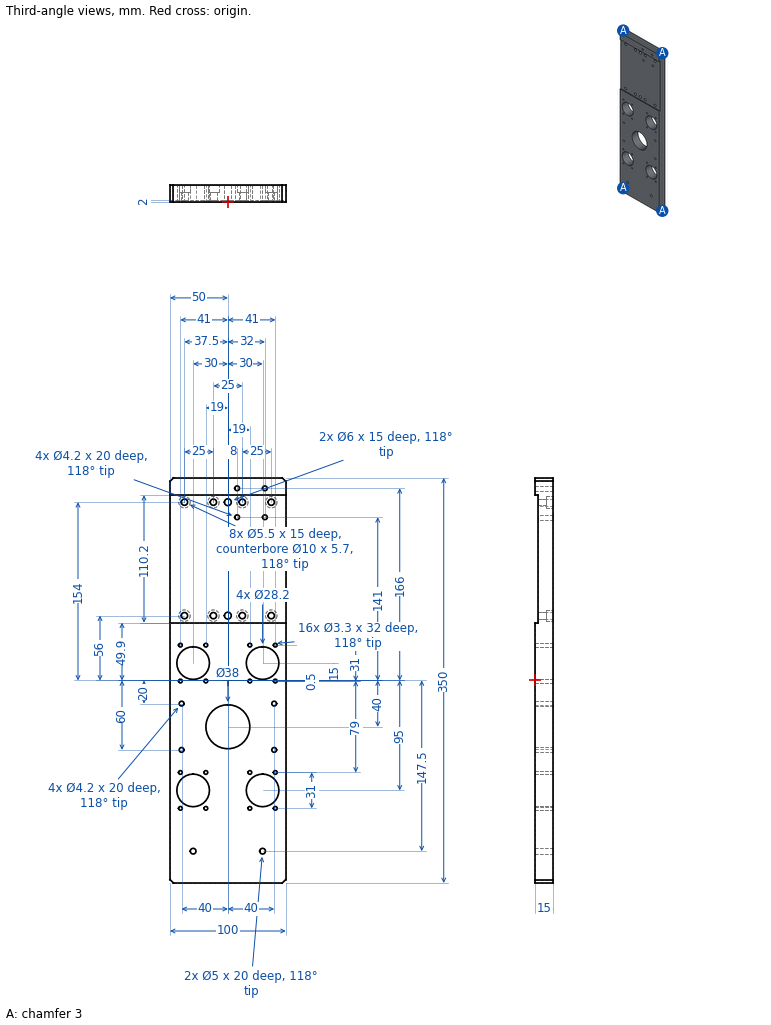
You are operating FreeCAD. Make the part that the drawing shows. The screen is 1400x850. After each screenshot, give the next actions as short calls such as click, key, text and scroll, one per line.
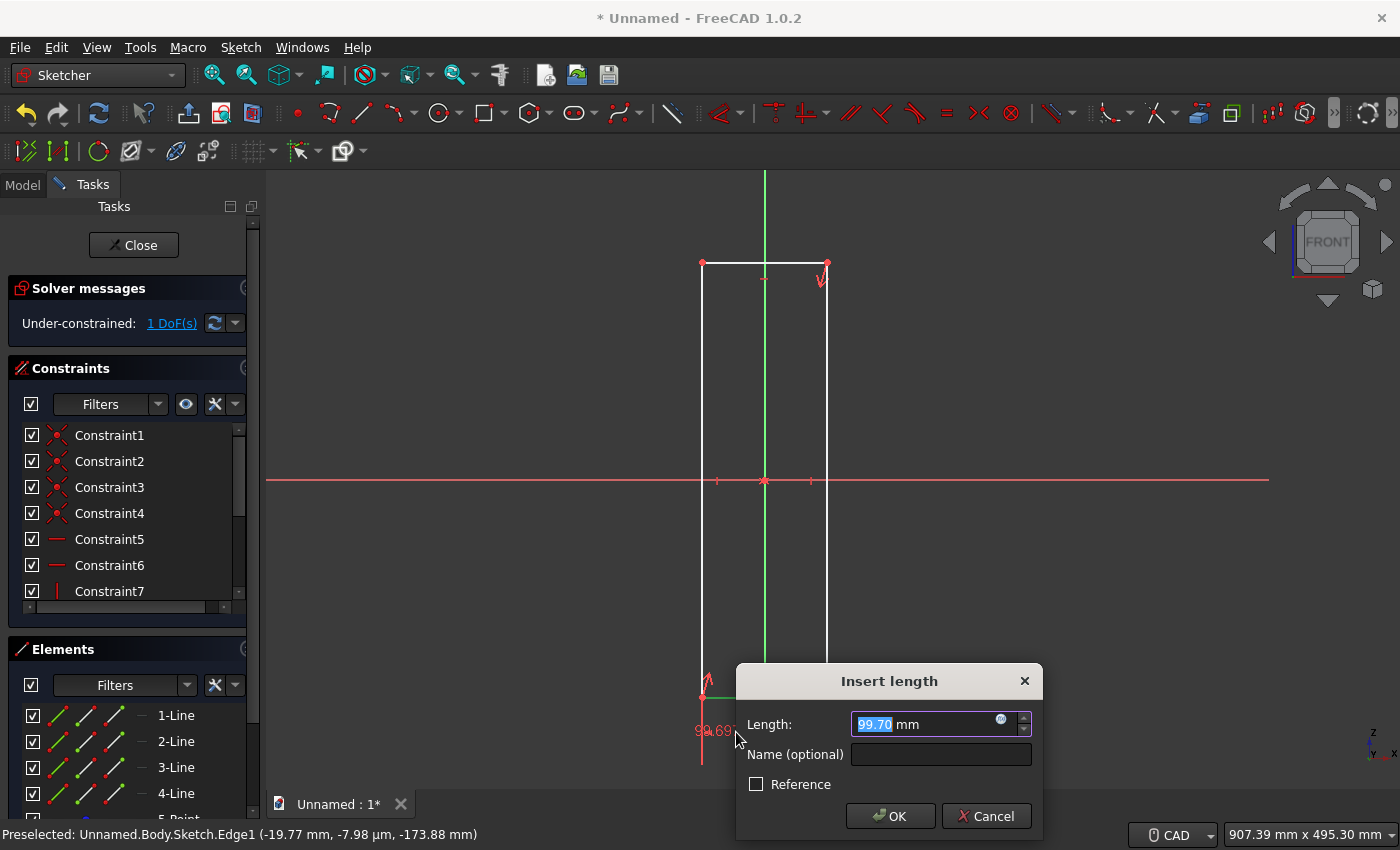
text(100)
key(Return)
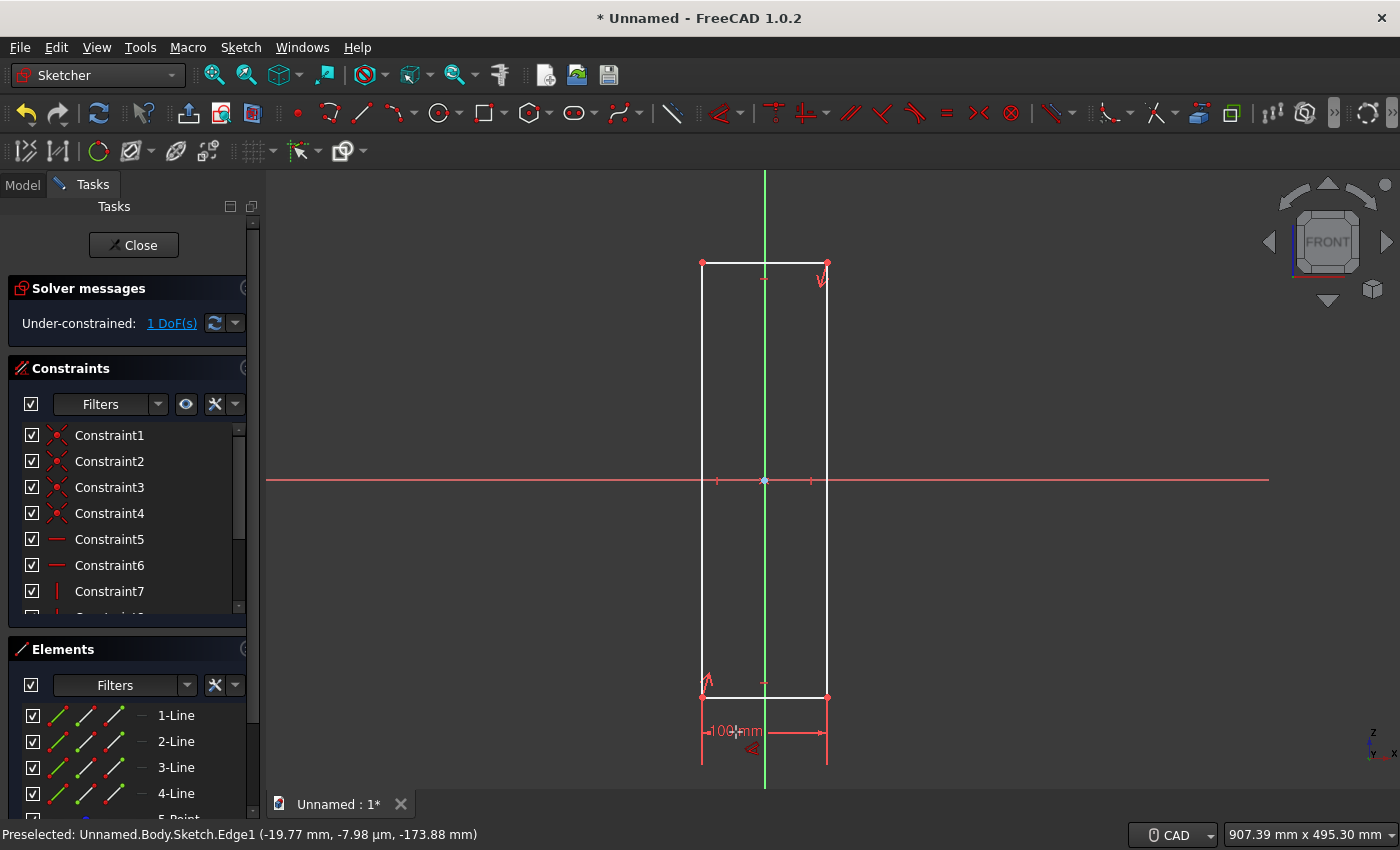
click(827, 567)
click(861, 380)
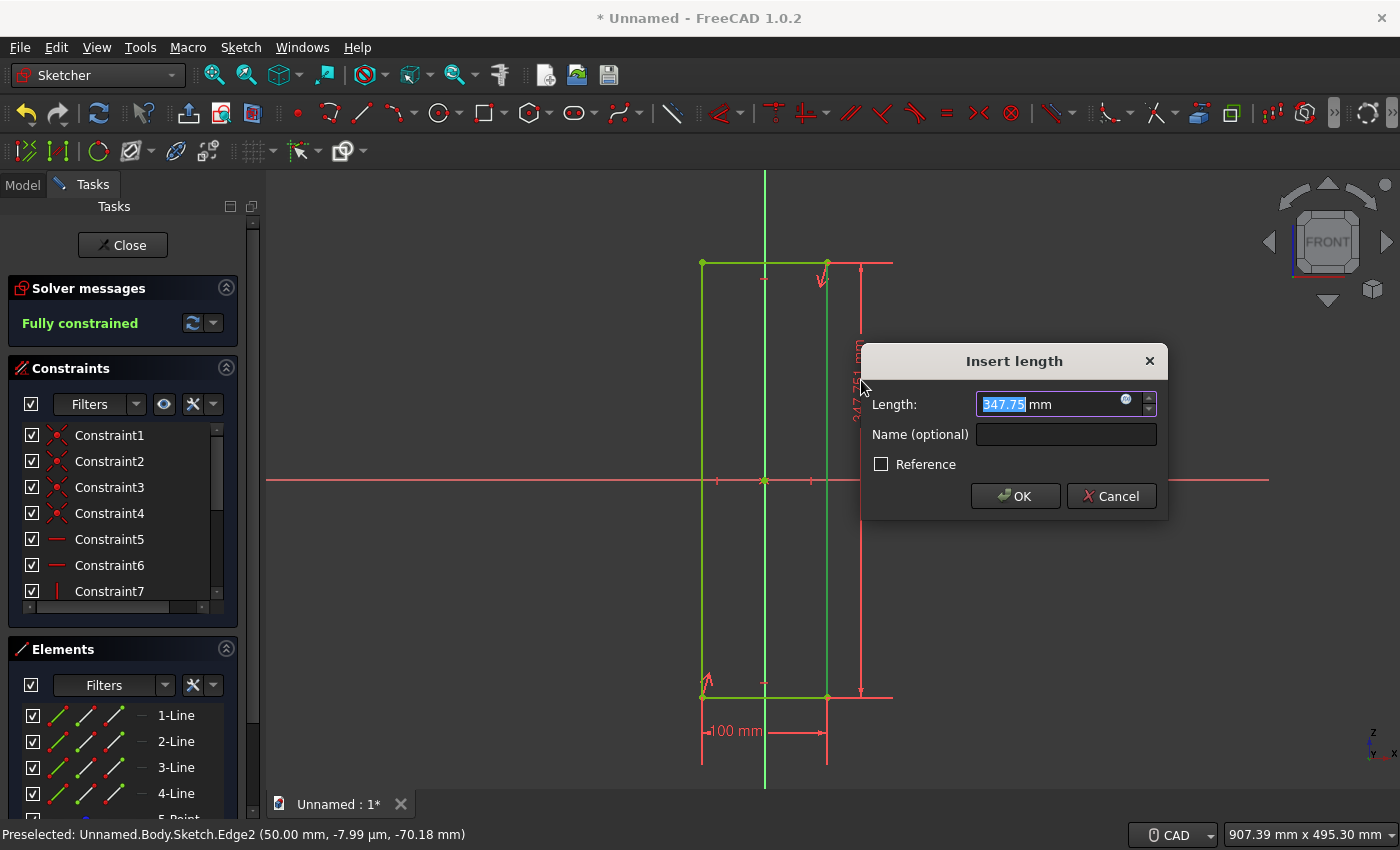
text(350)
key(Return)
key(Escape)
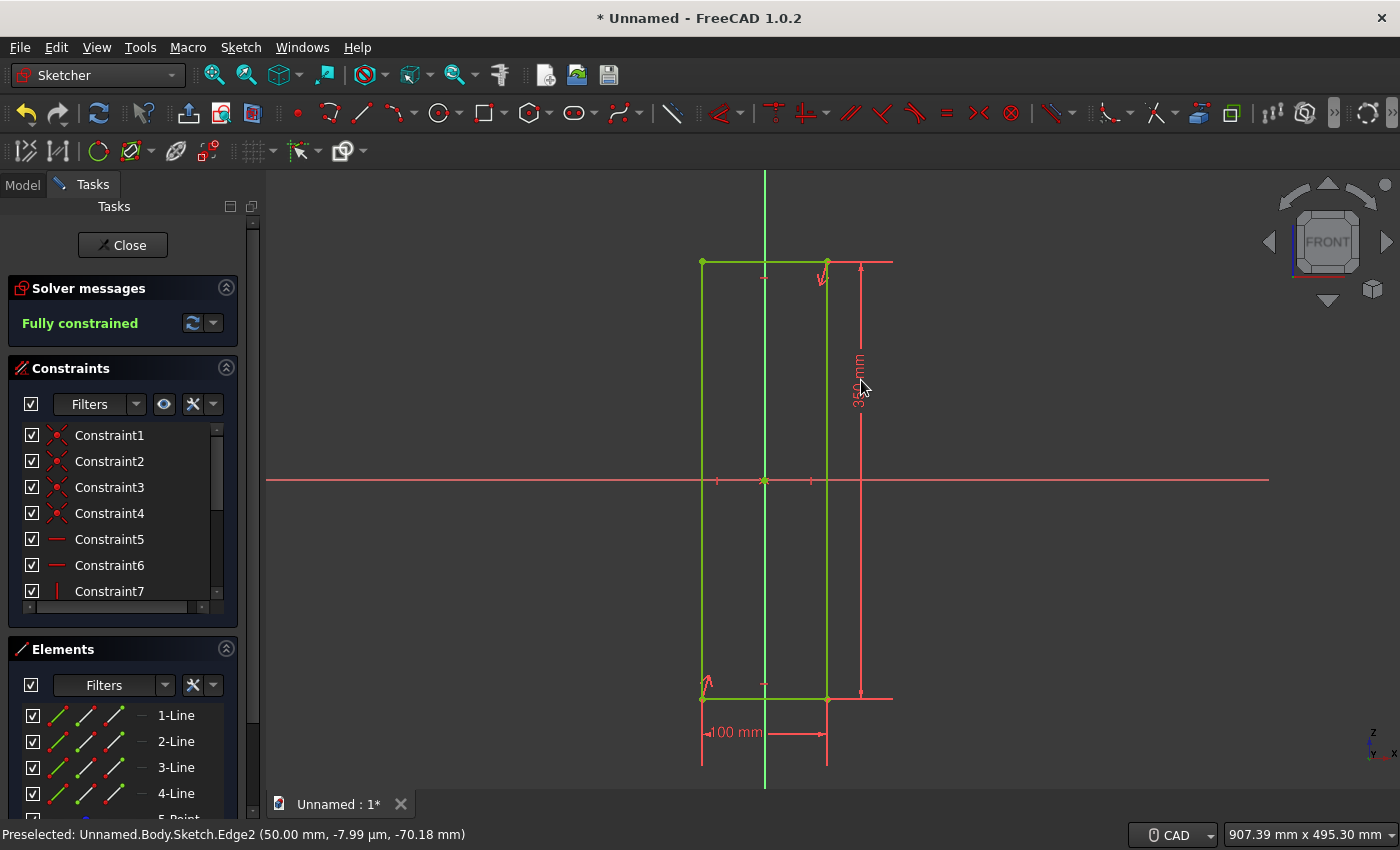
click(123, 245)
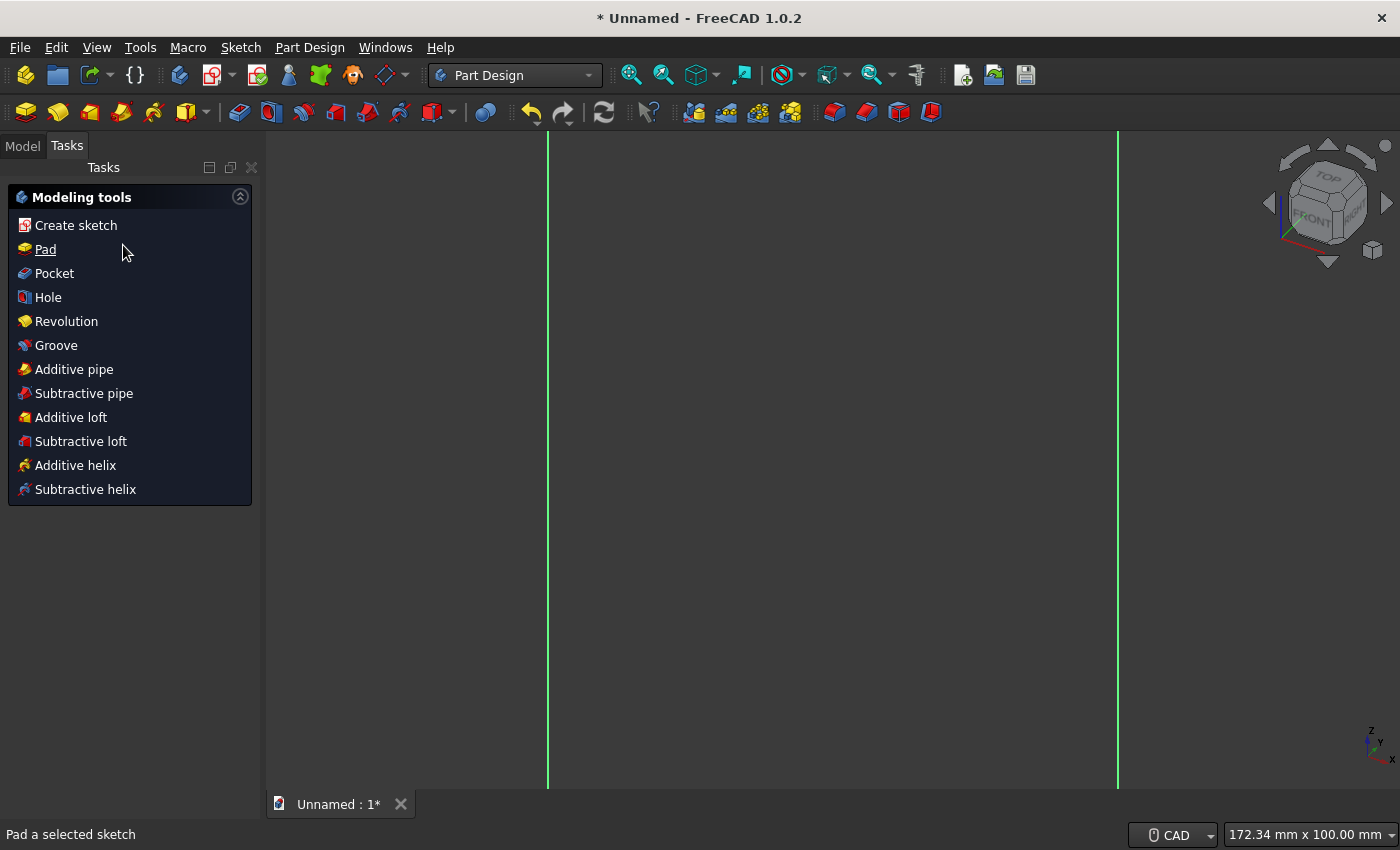
click(26, 112)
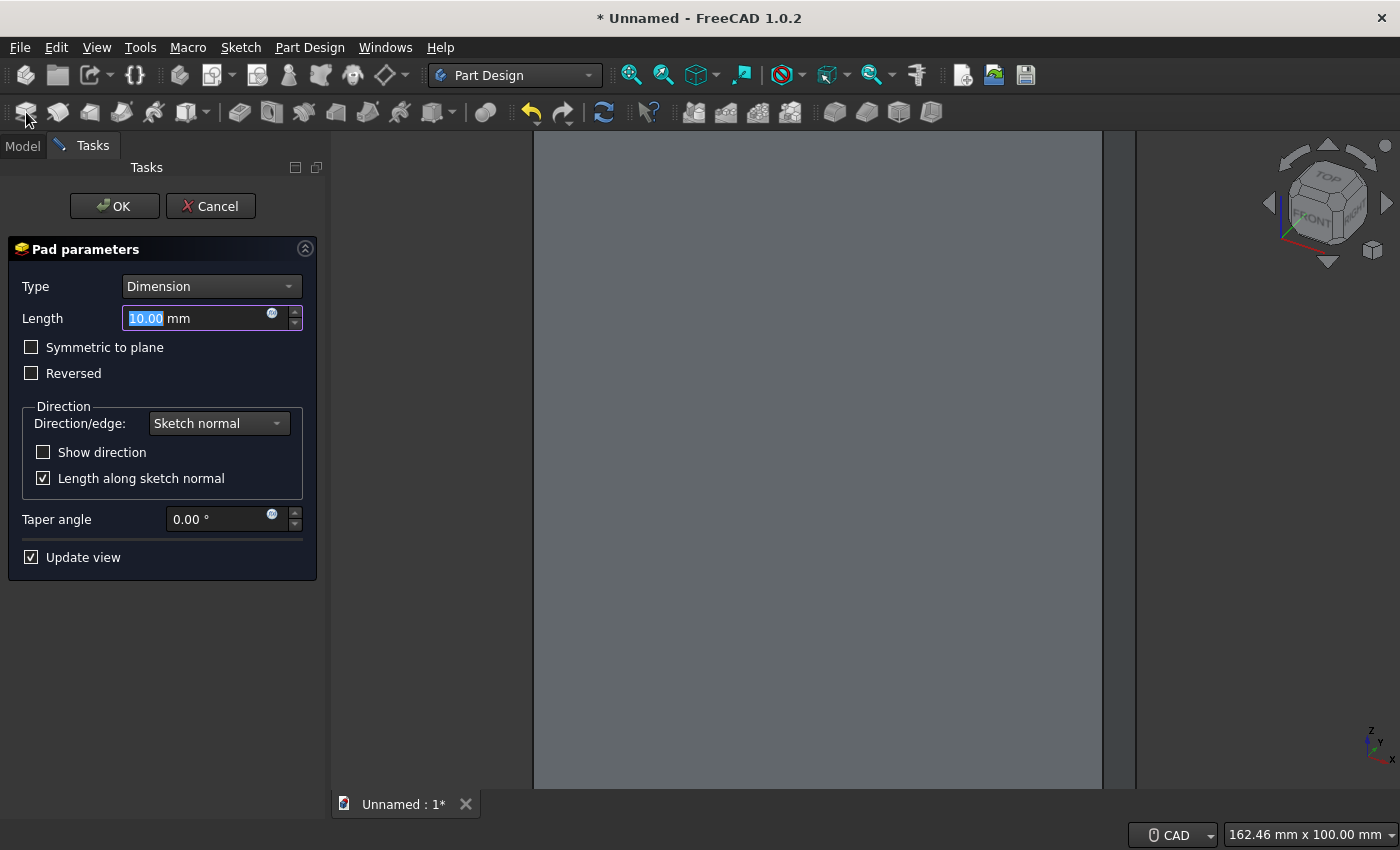
text(15)
key(Tab)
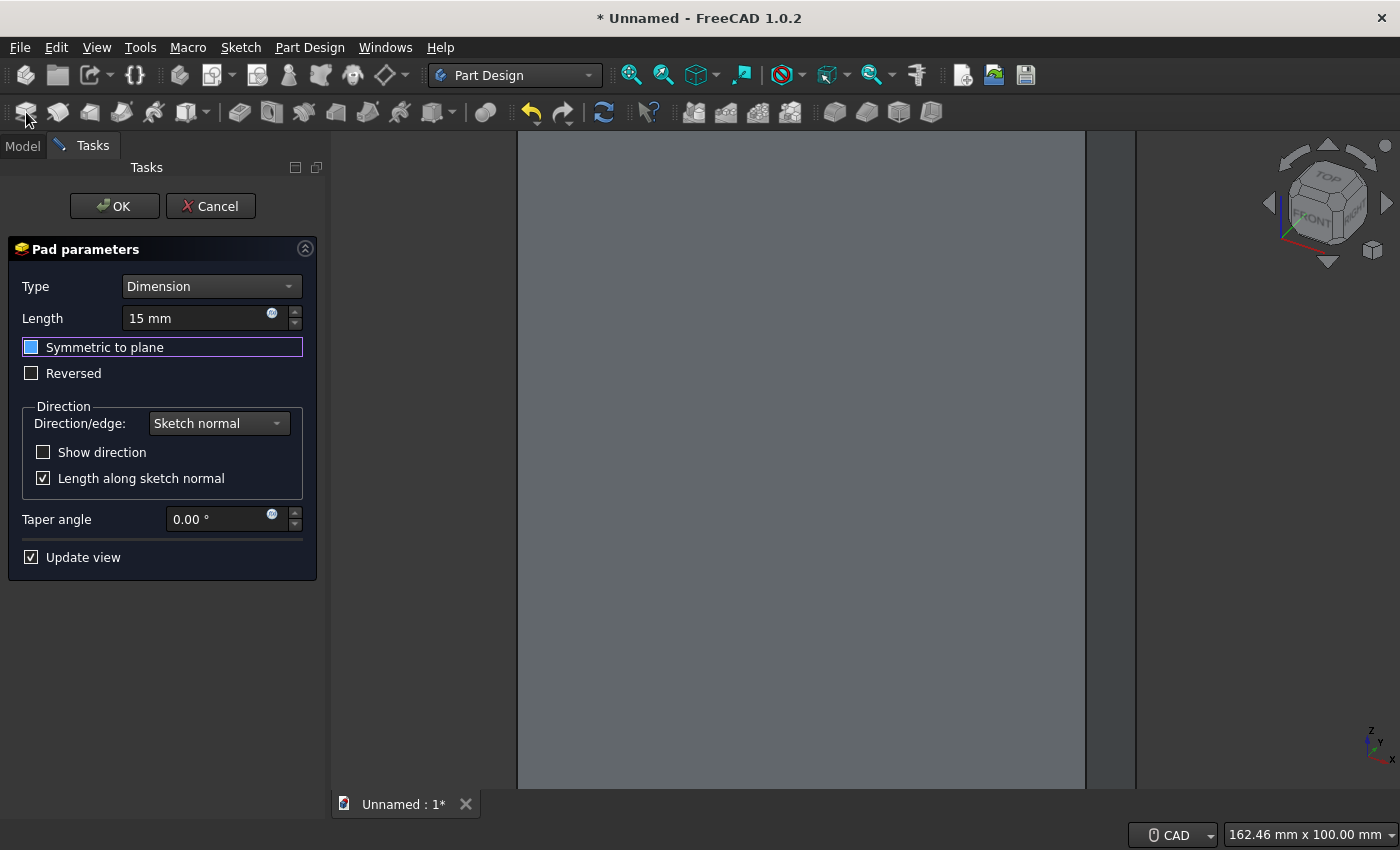
click(30, 373)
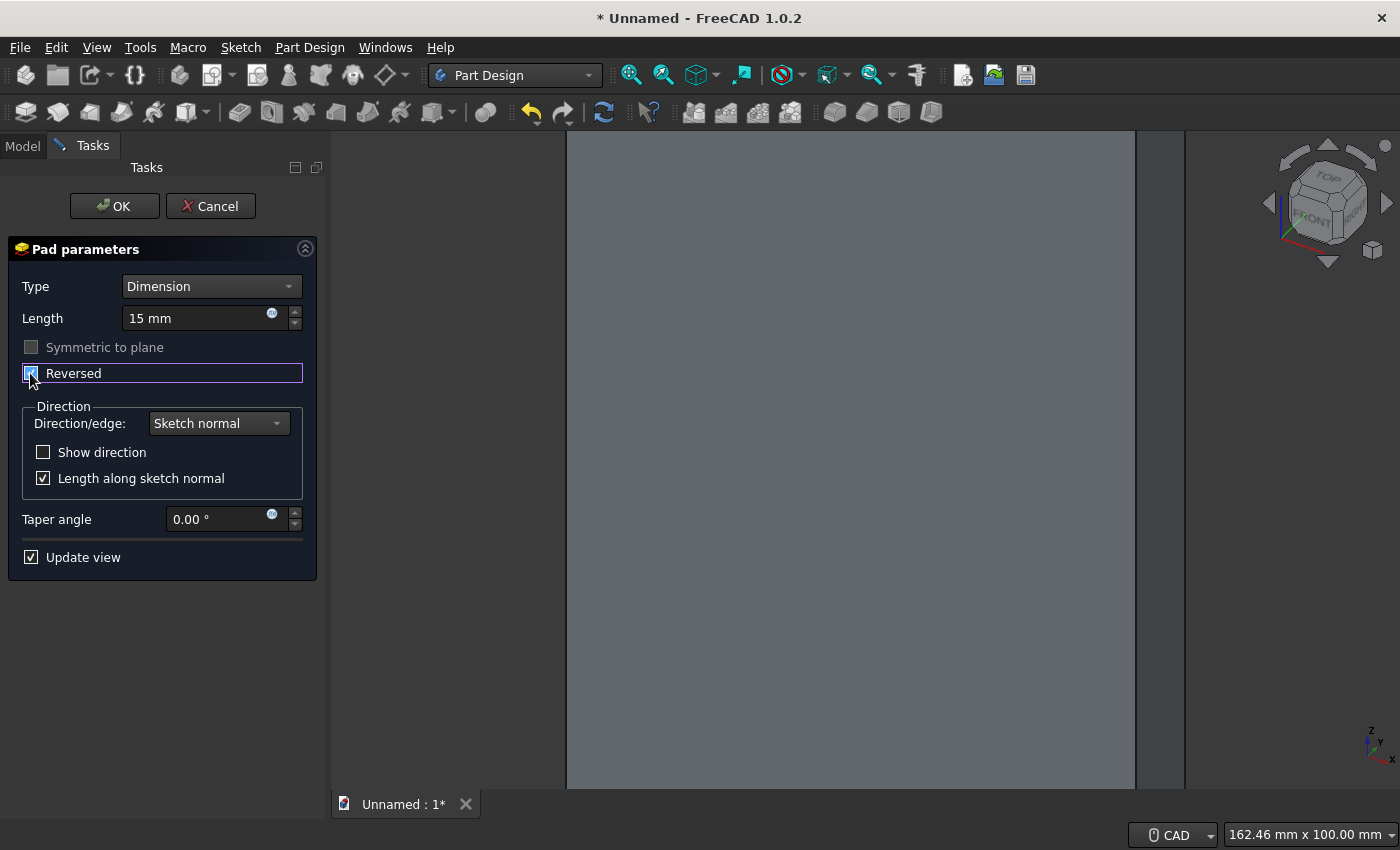
click(115, 206)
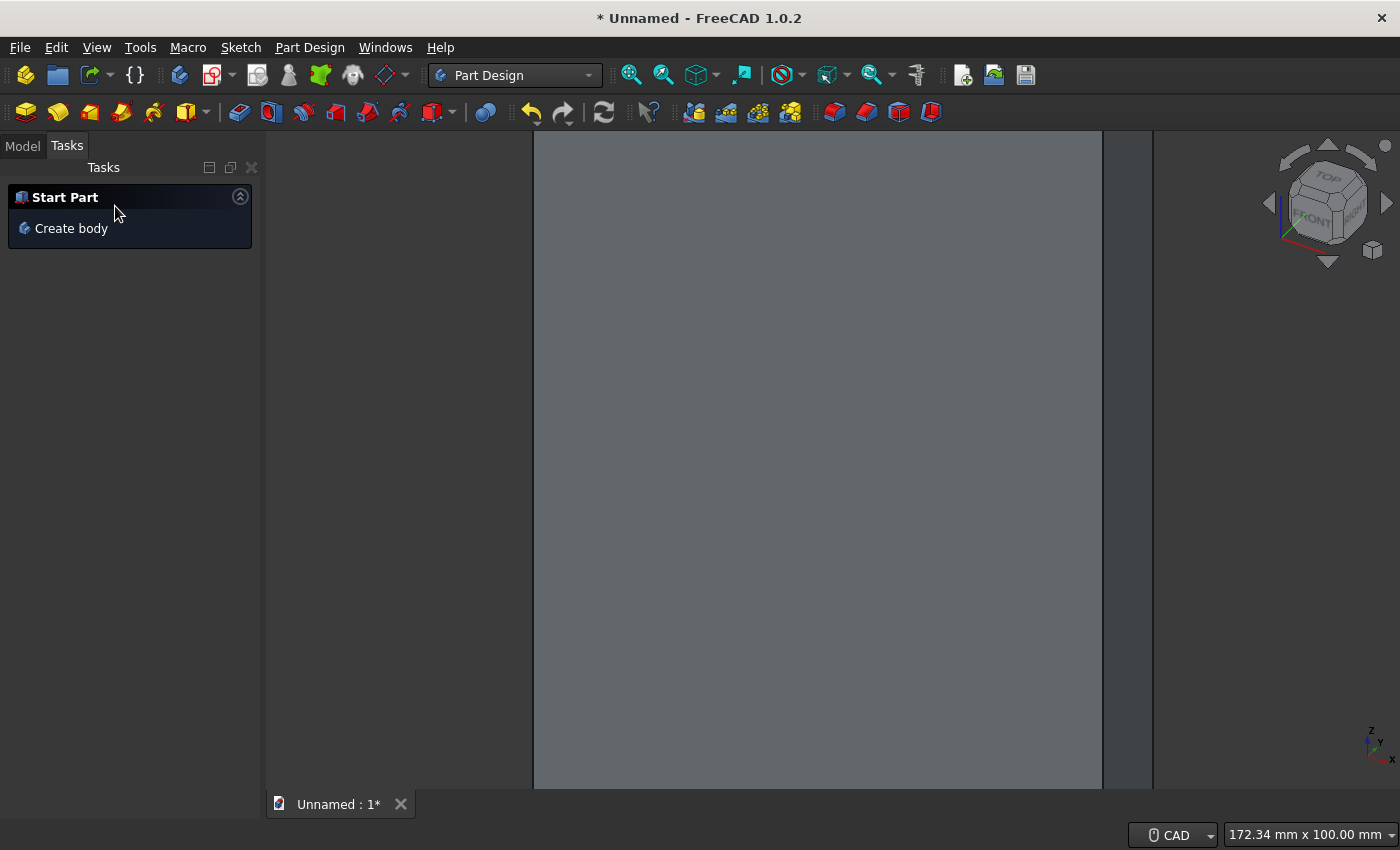
click(632, 76)